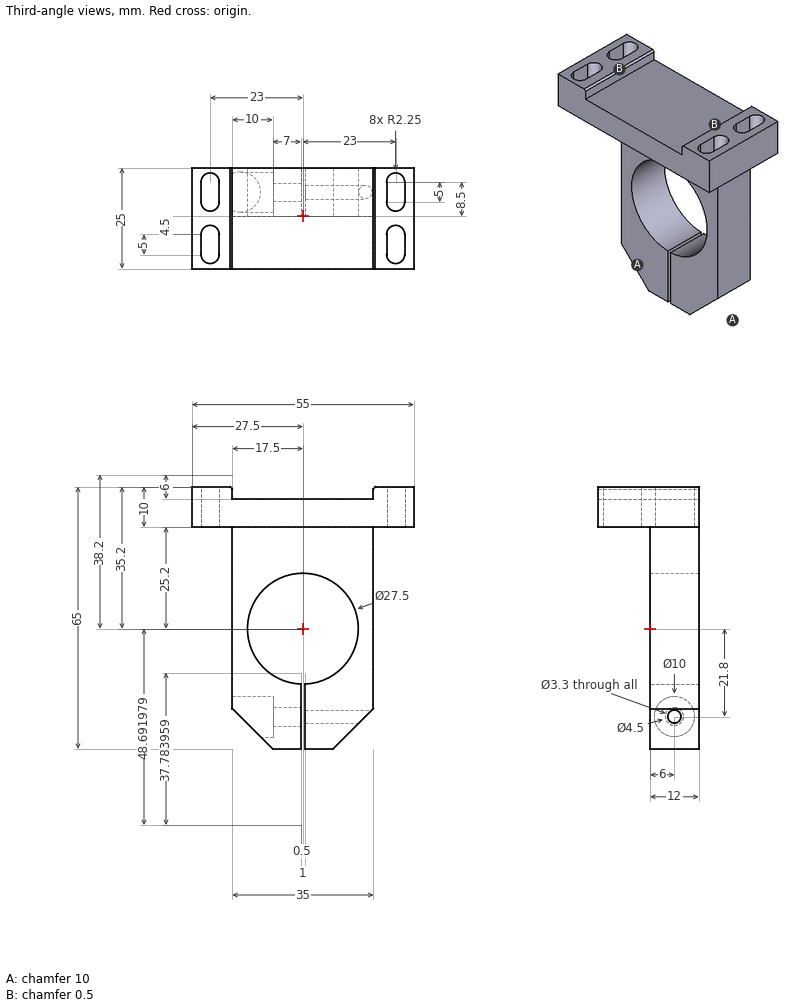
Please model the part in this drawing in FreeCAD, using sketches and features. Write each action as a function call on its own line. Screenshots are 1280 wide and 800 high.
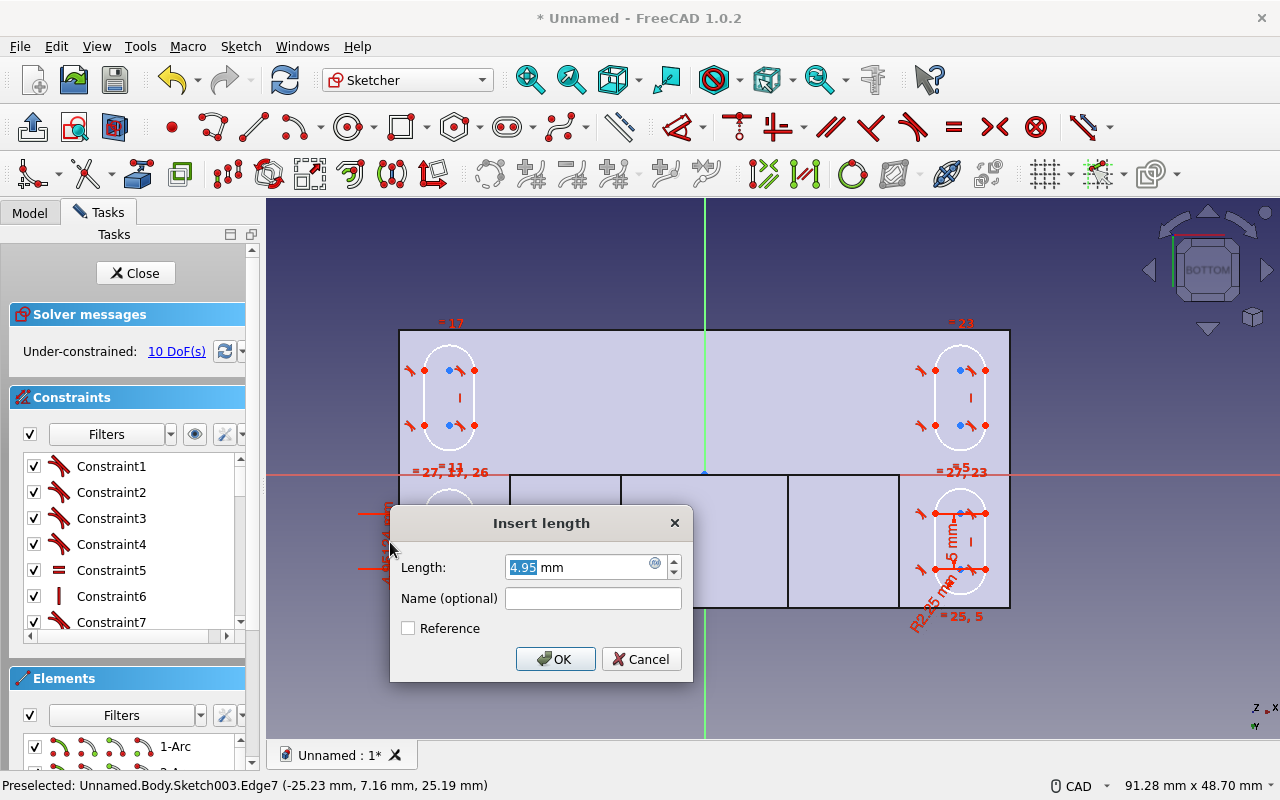
text(5)
key(Return)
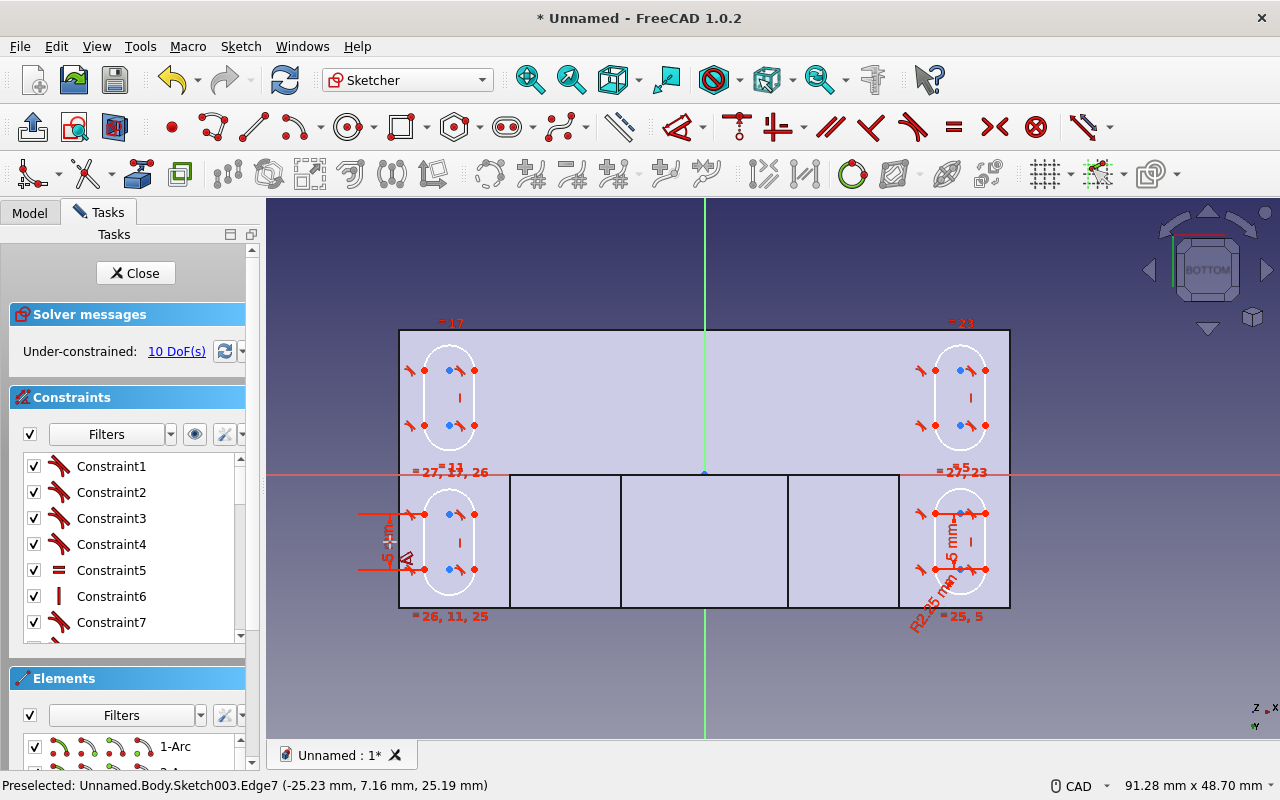
click(424, 409)
click(390, 398)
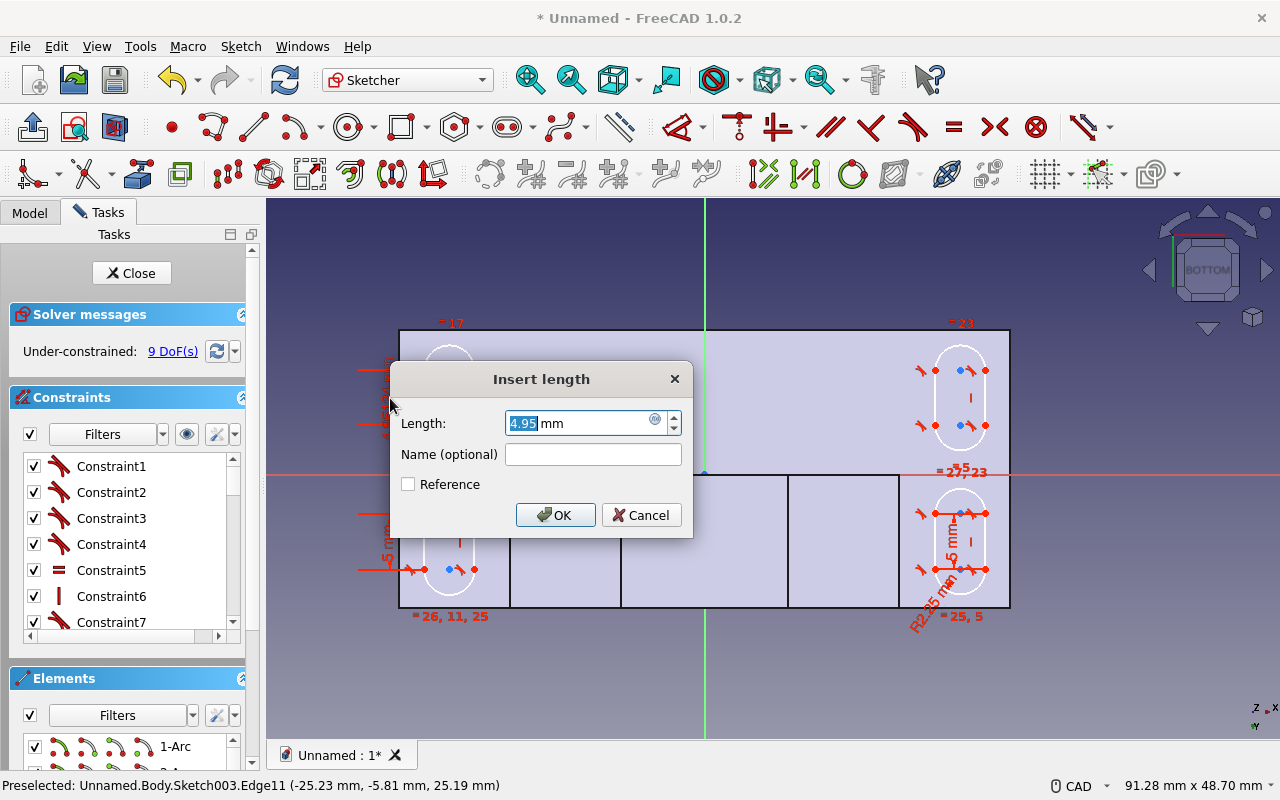
text(5)
key(Return)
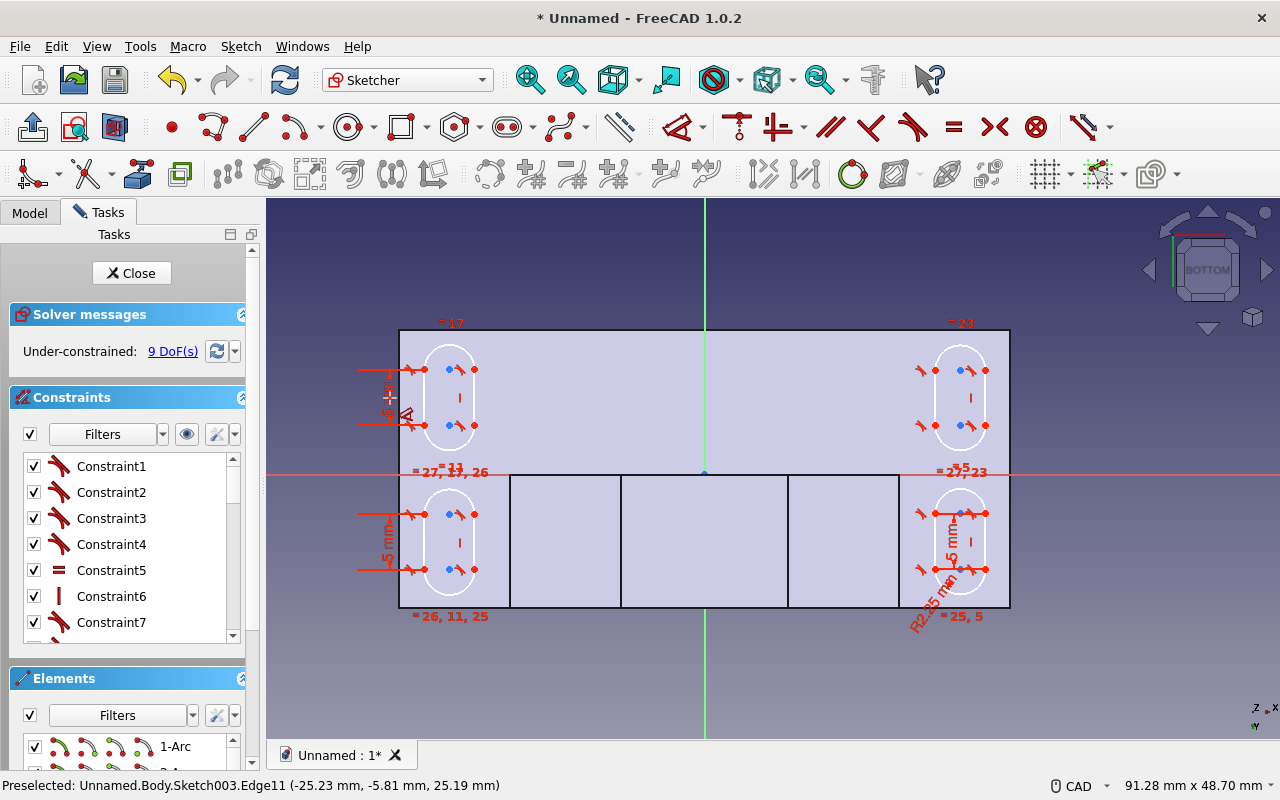
click(935, 409)
click(969, 398)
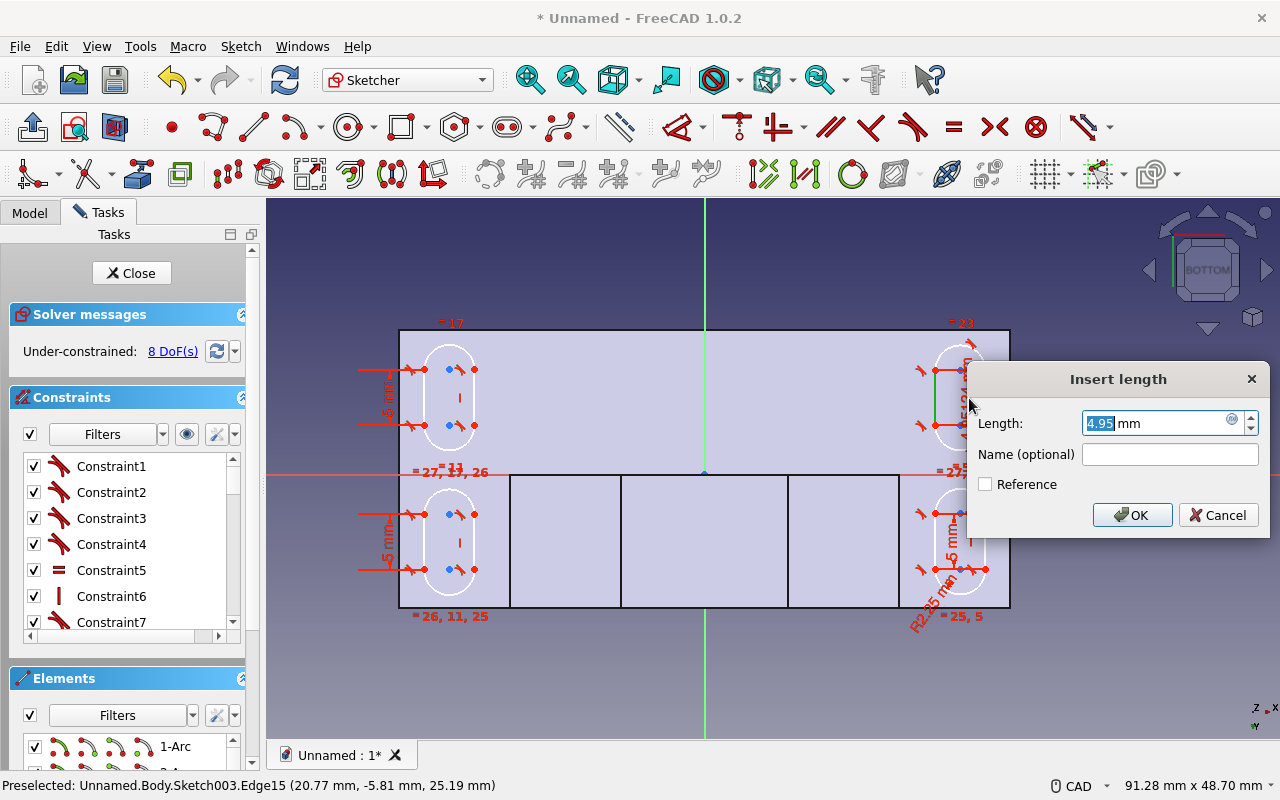
text(5)
key(Return)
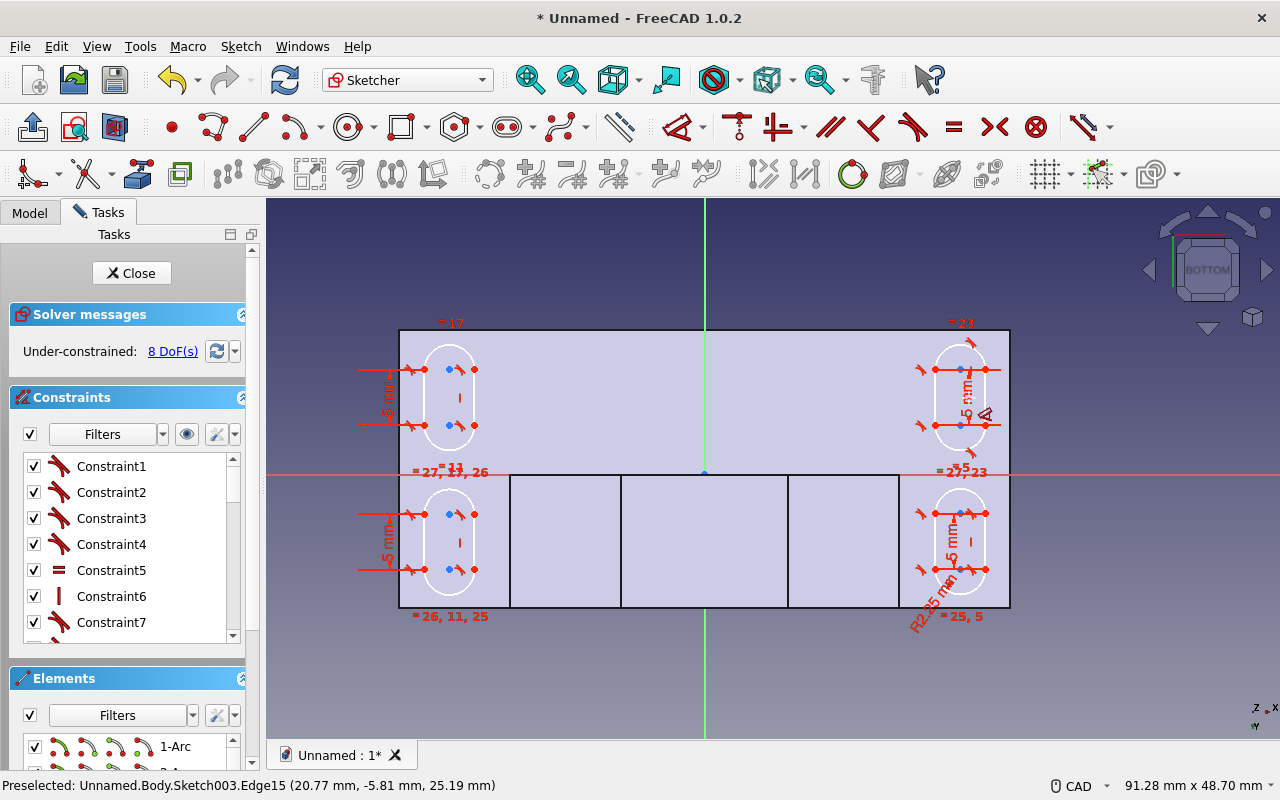
click(960, 569)
click(833, 603)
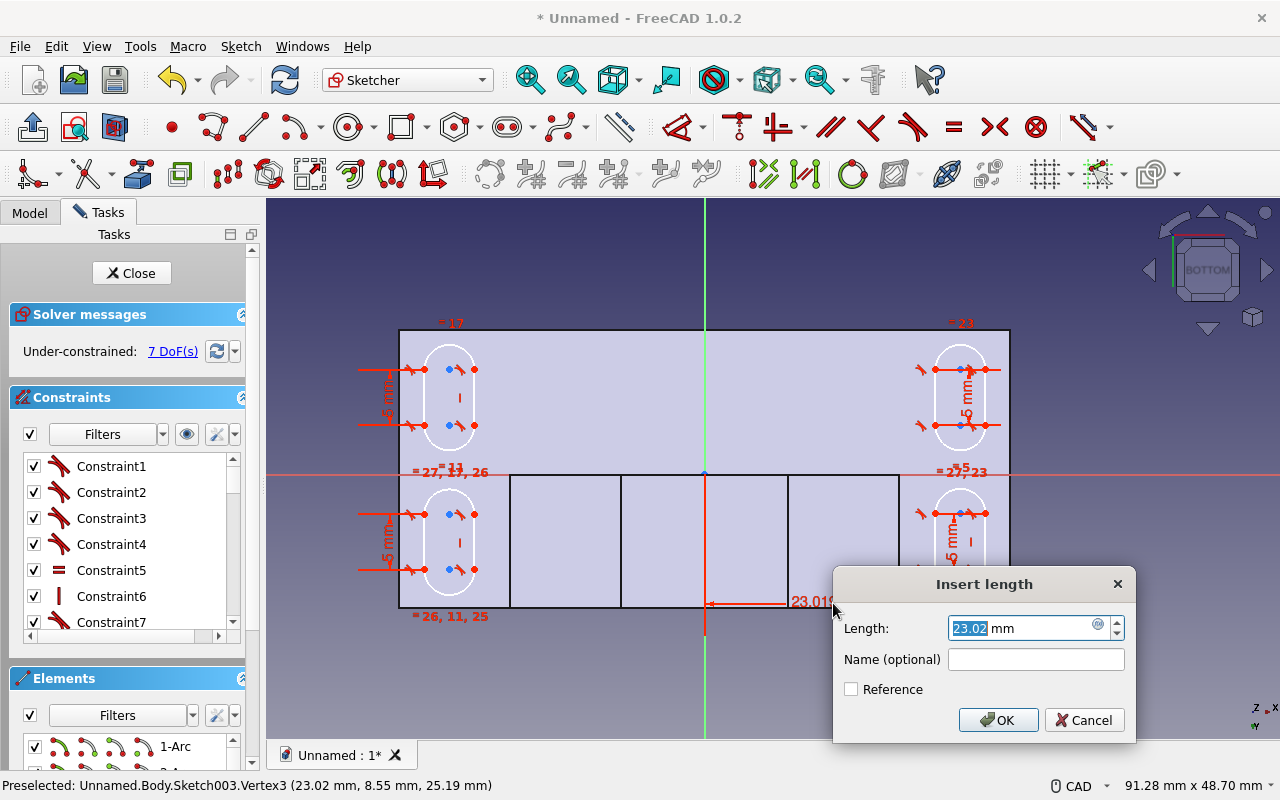
text(23)
key(Return)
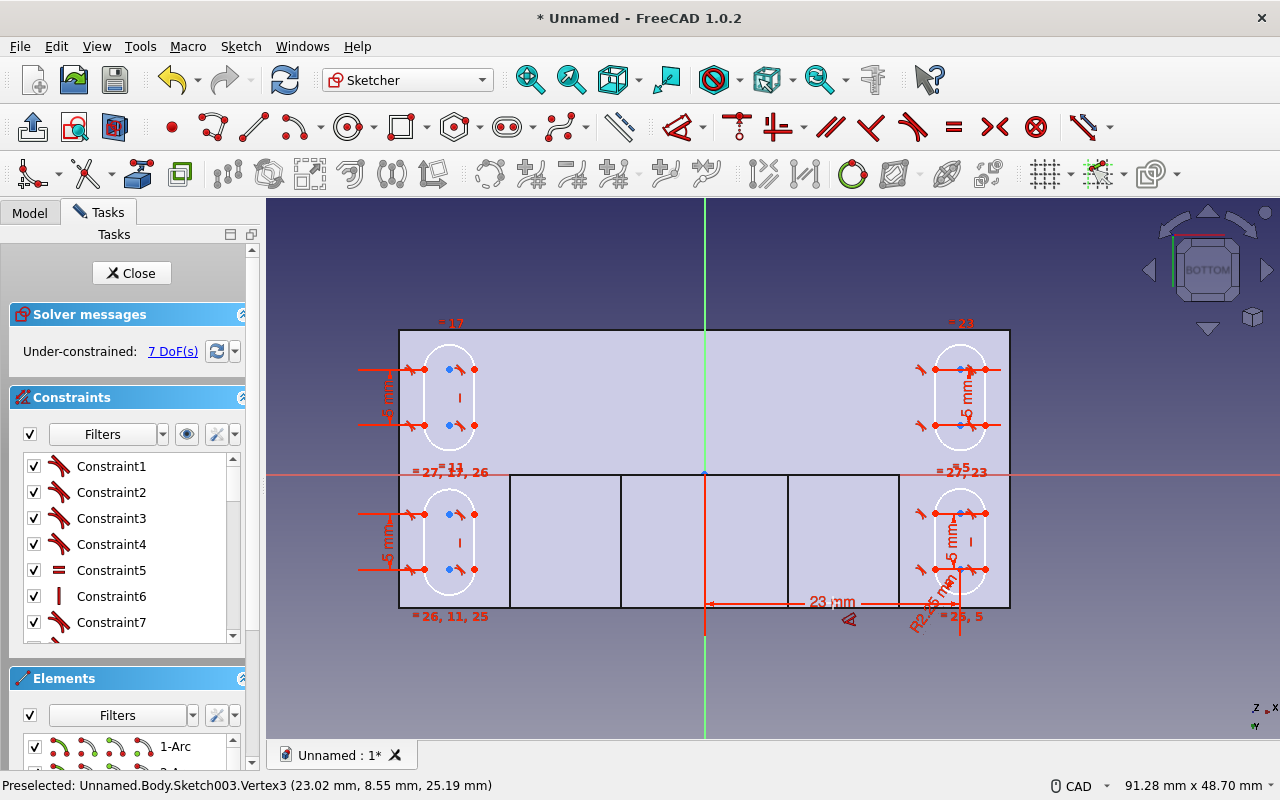
click(449, 570)
click(577, 604)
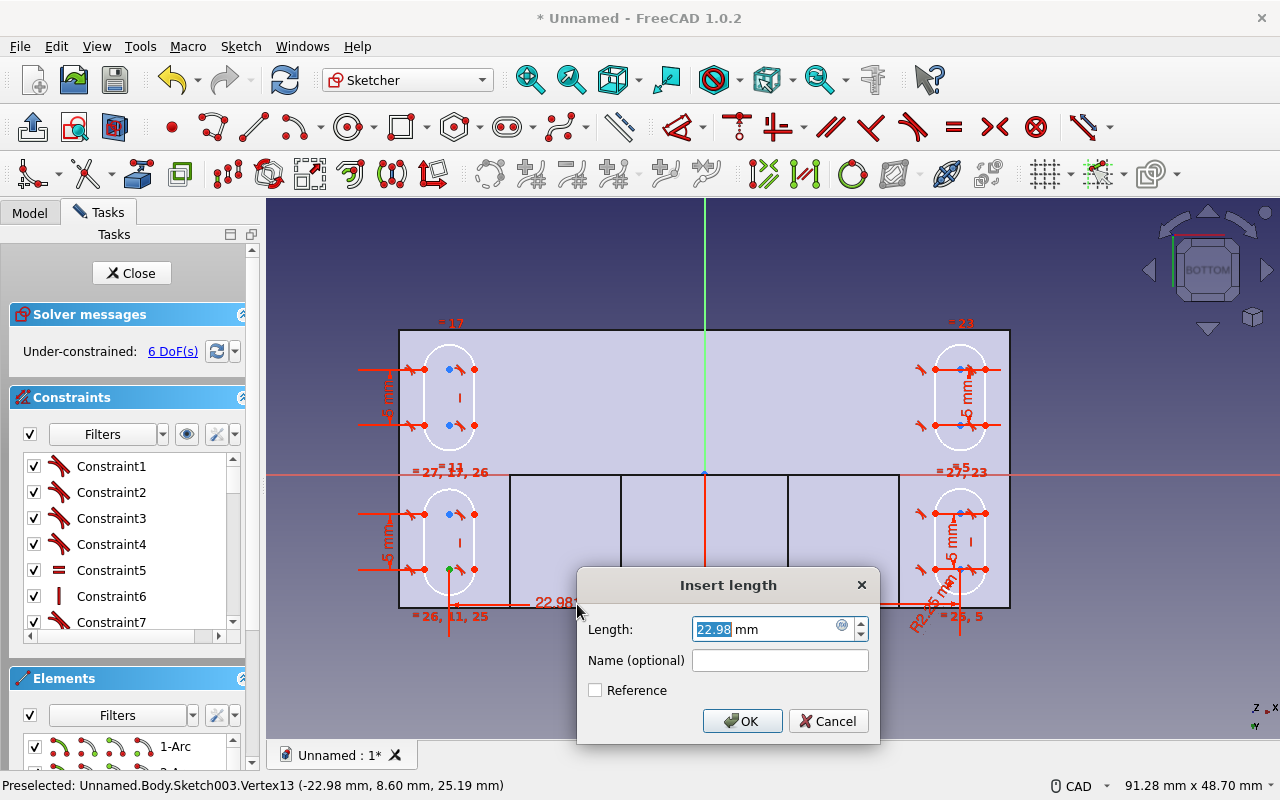
text(23)
key(Return)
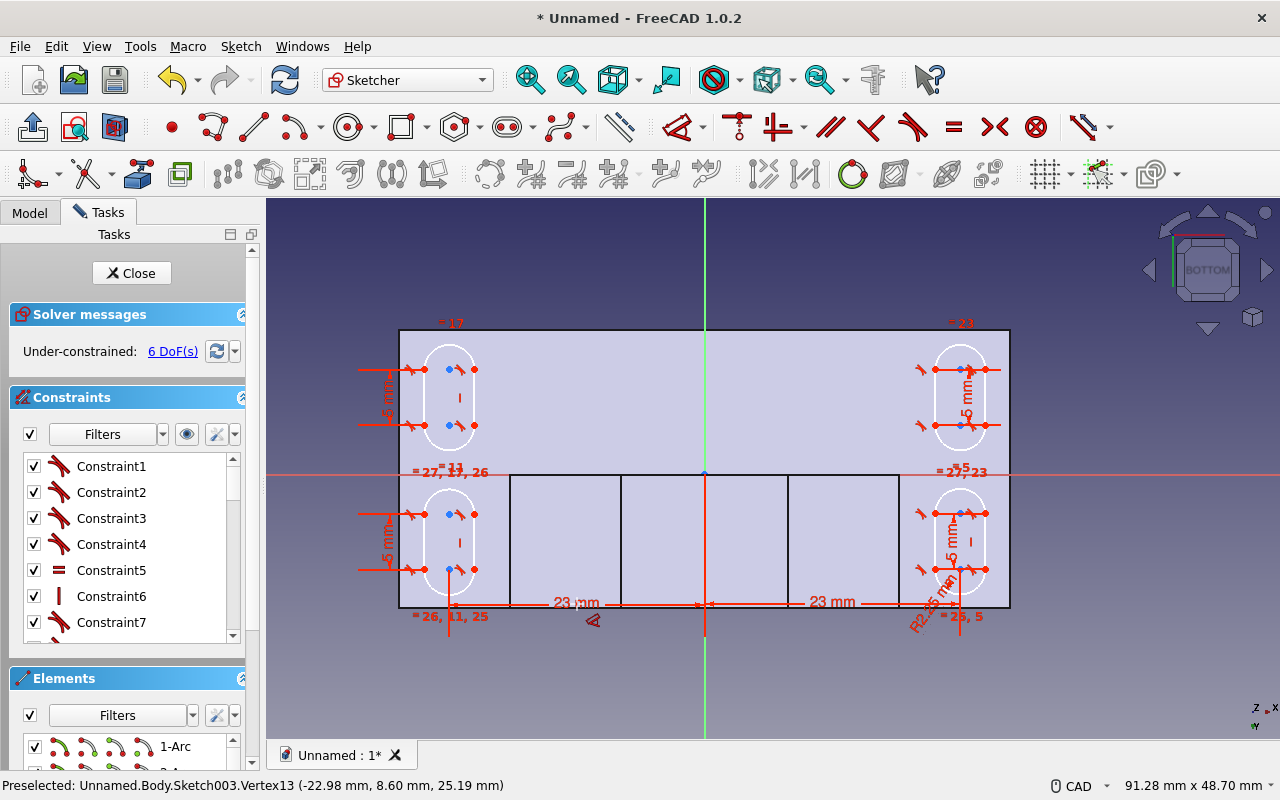
click(449, 425)
click(577, 391)